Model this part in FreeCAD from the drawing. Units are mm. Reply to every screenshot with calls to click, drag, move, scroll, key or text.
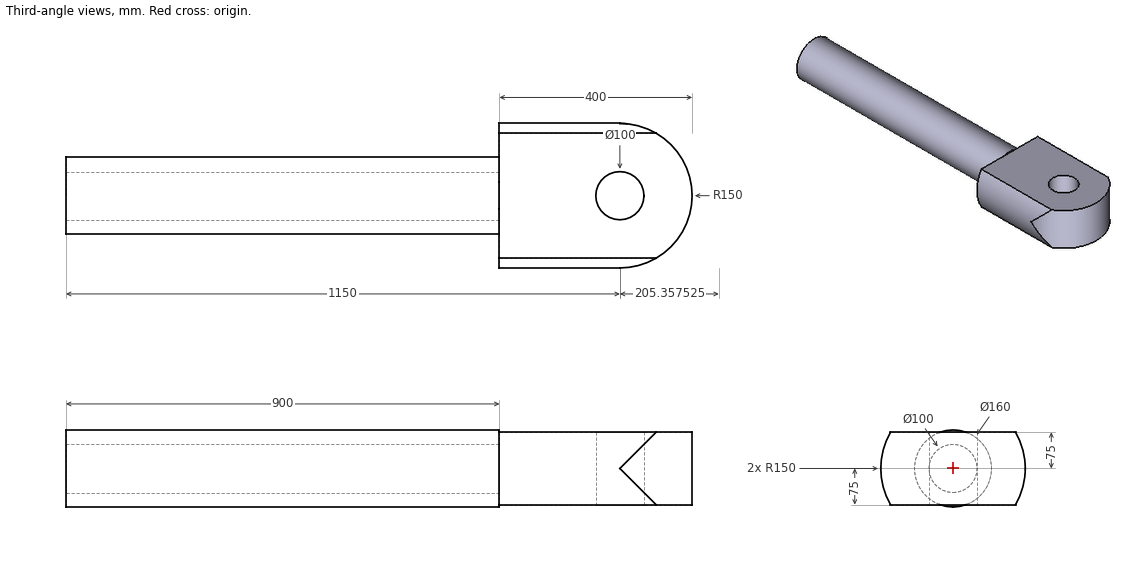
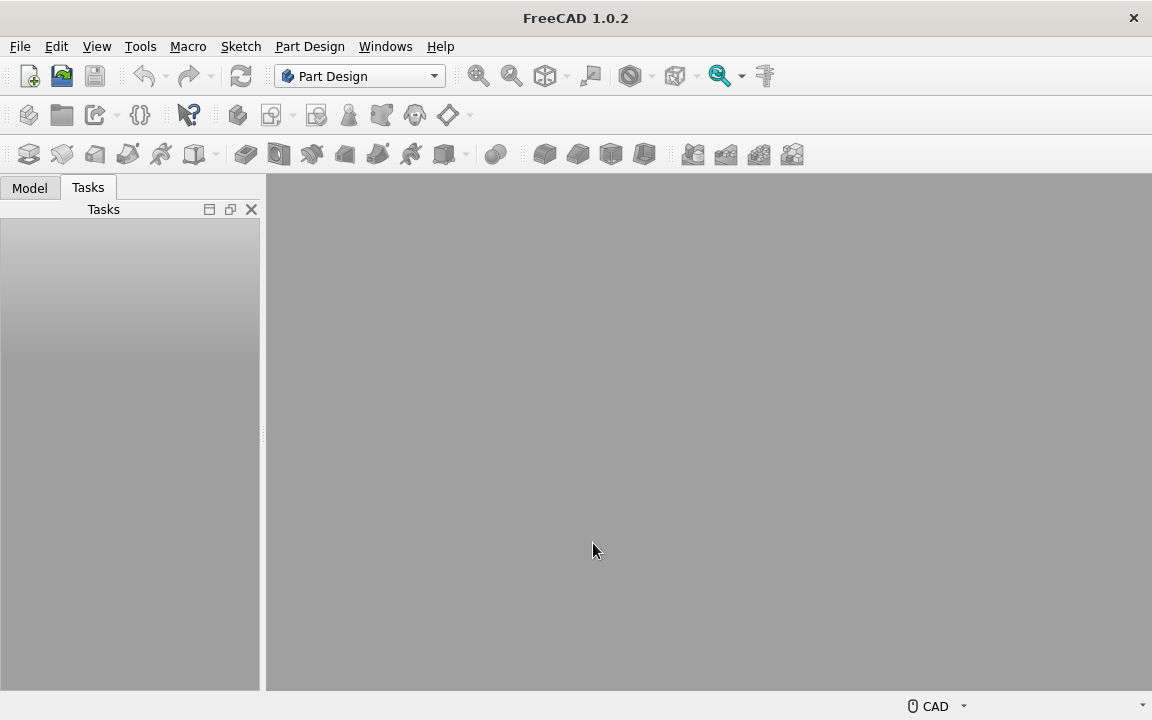
key(ctrl+n)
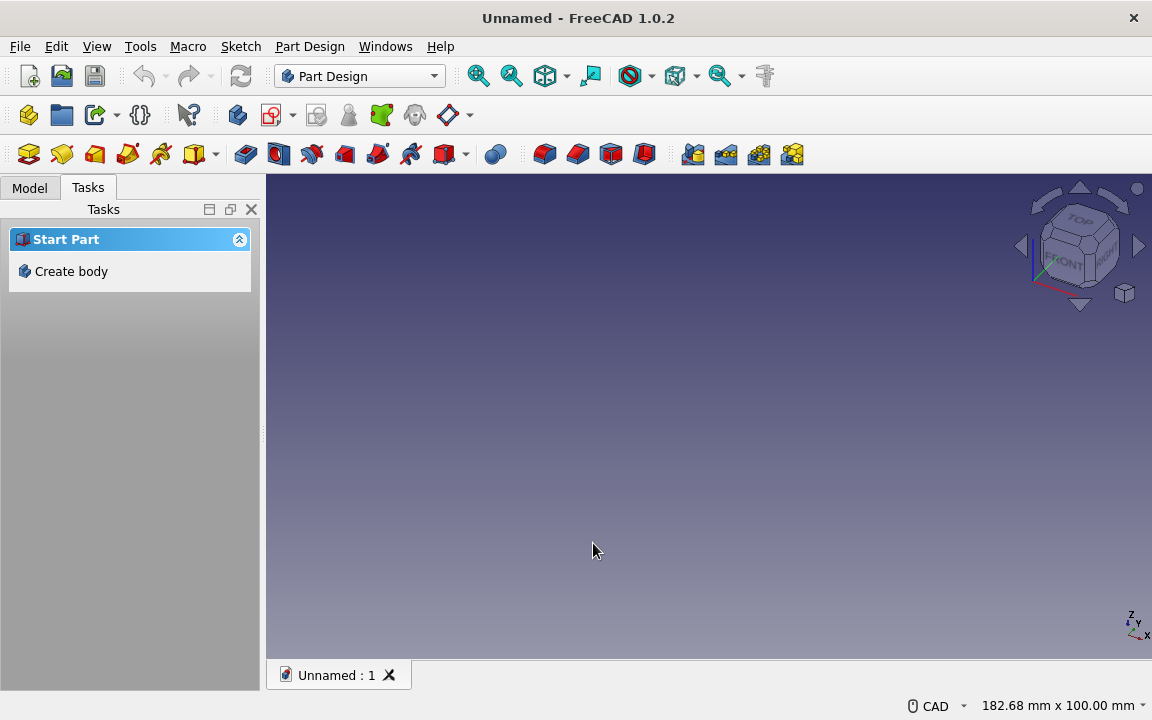
click(238, 116)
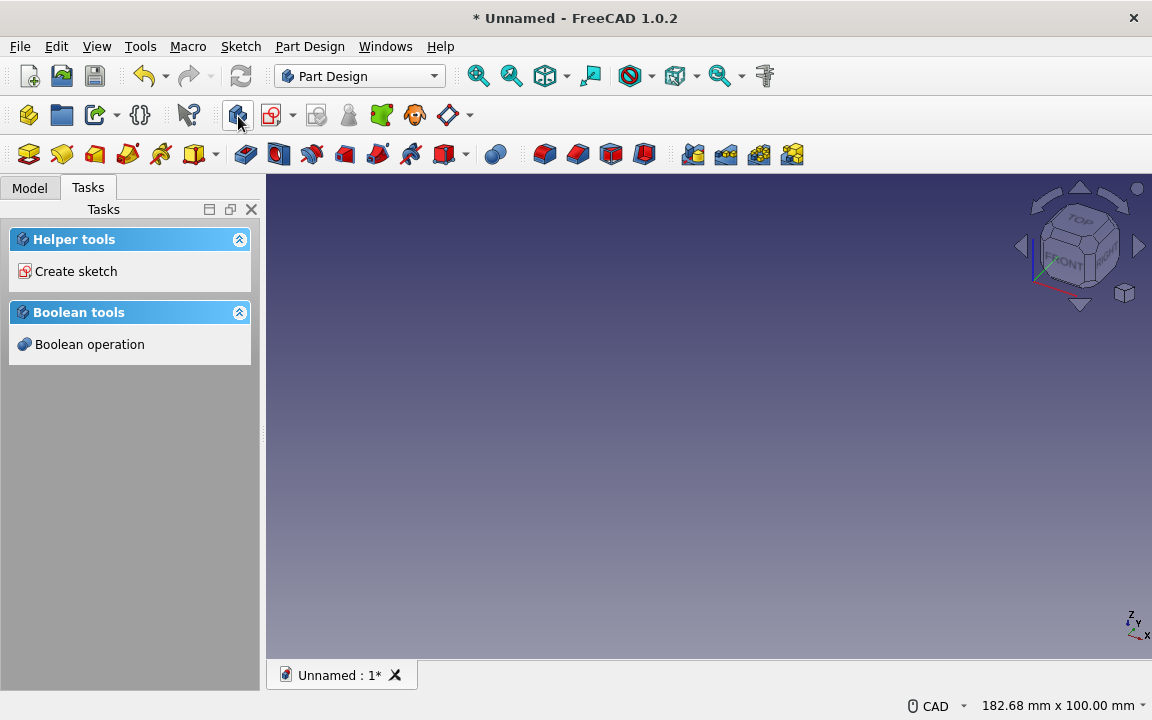
click(30, 188)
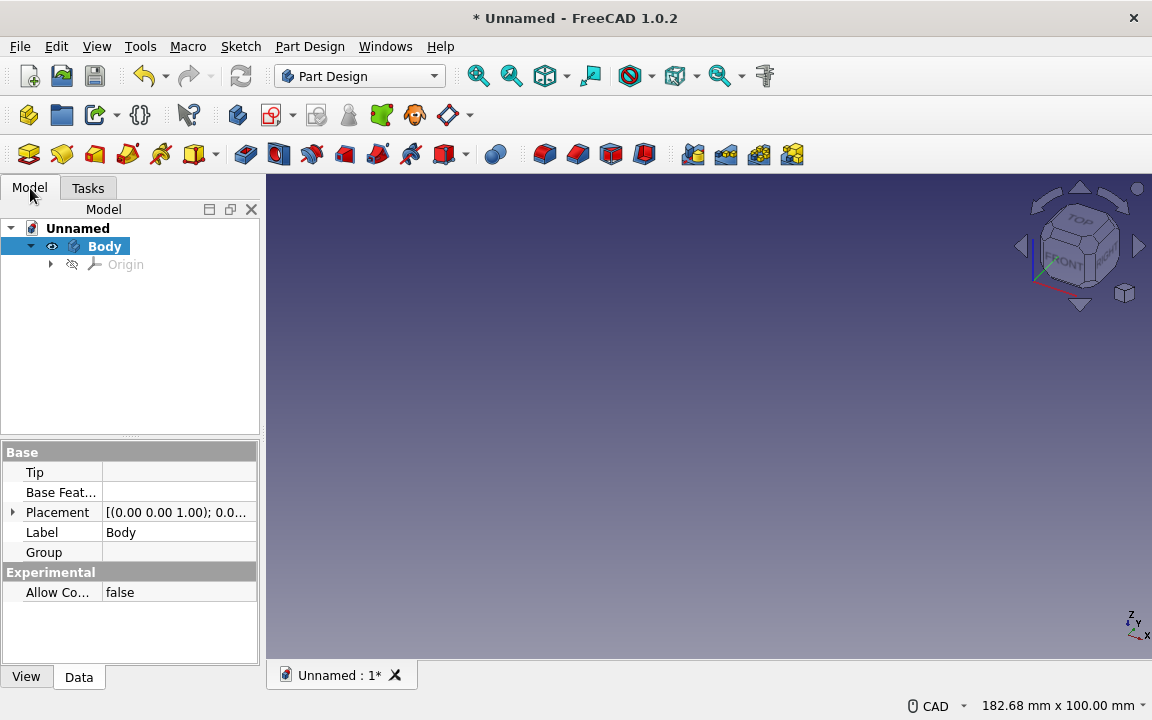
click(51, 264)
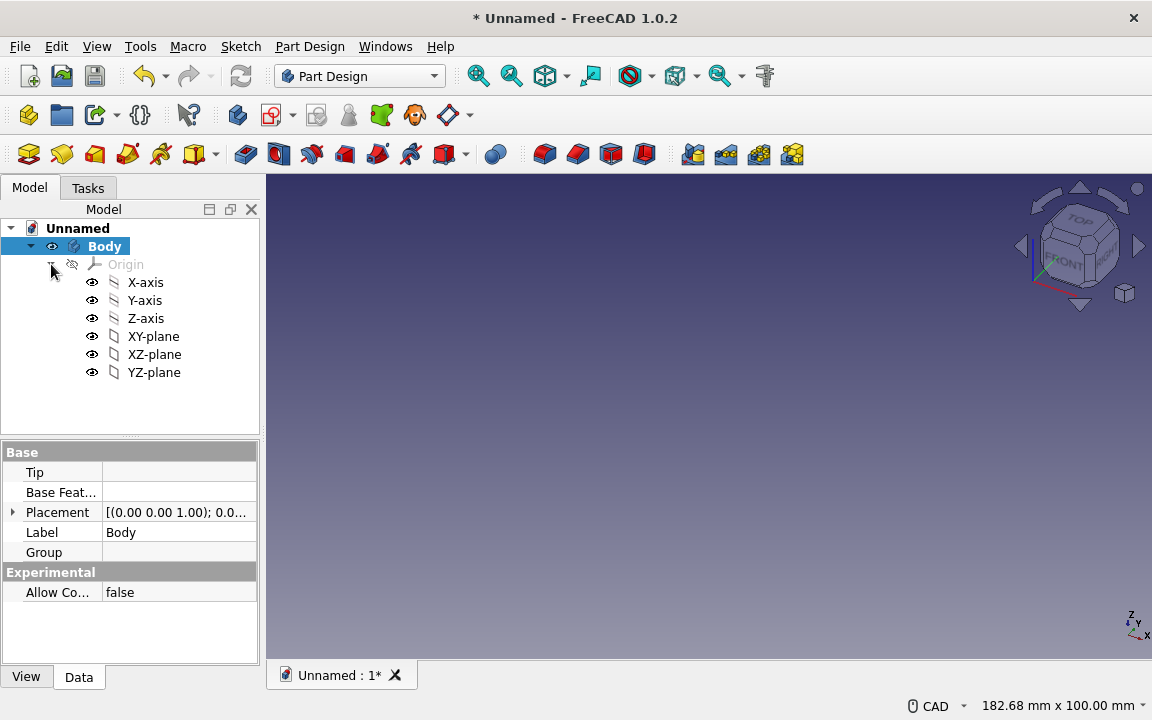
click(137, 372)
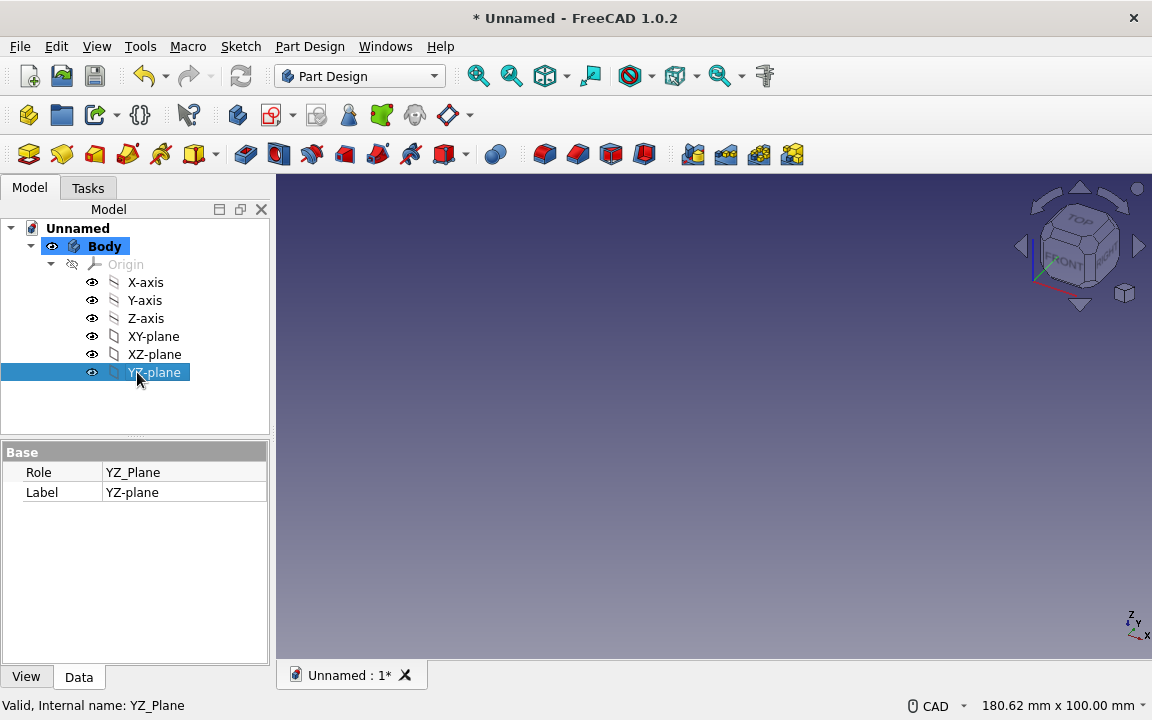
click(448, 116)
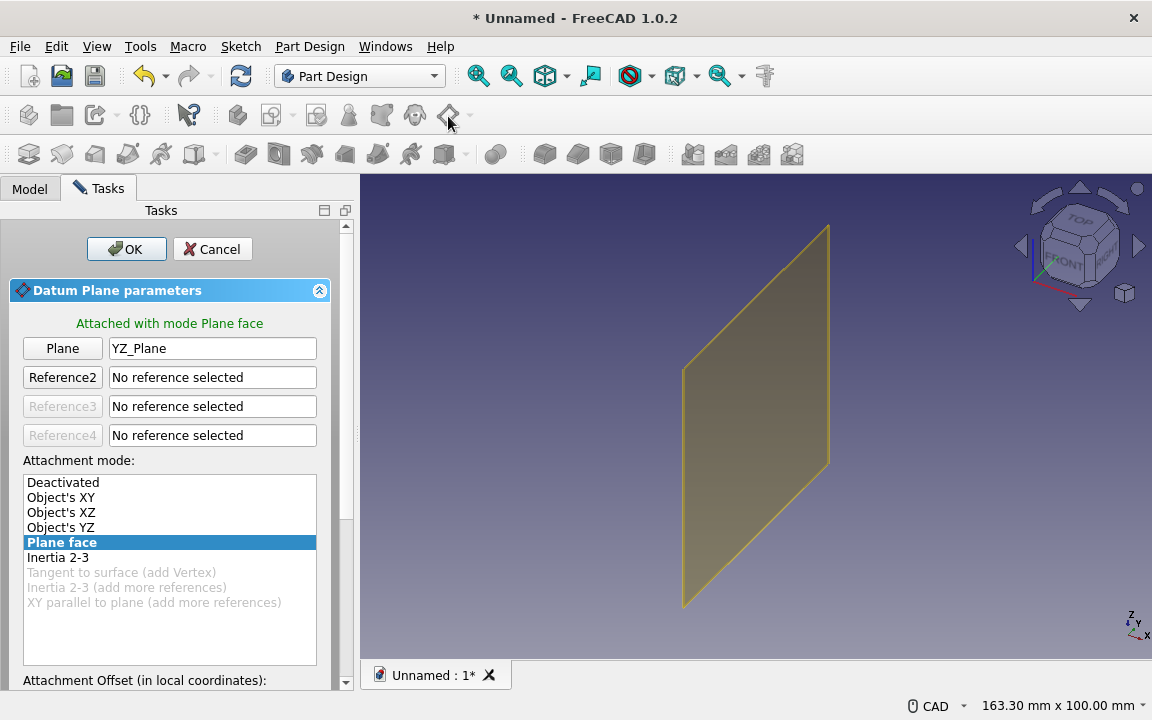
scroll(346, 455, down, 3)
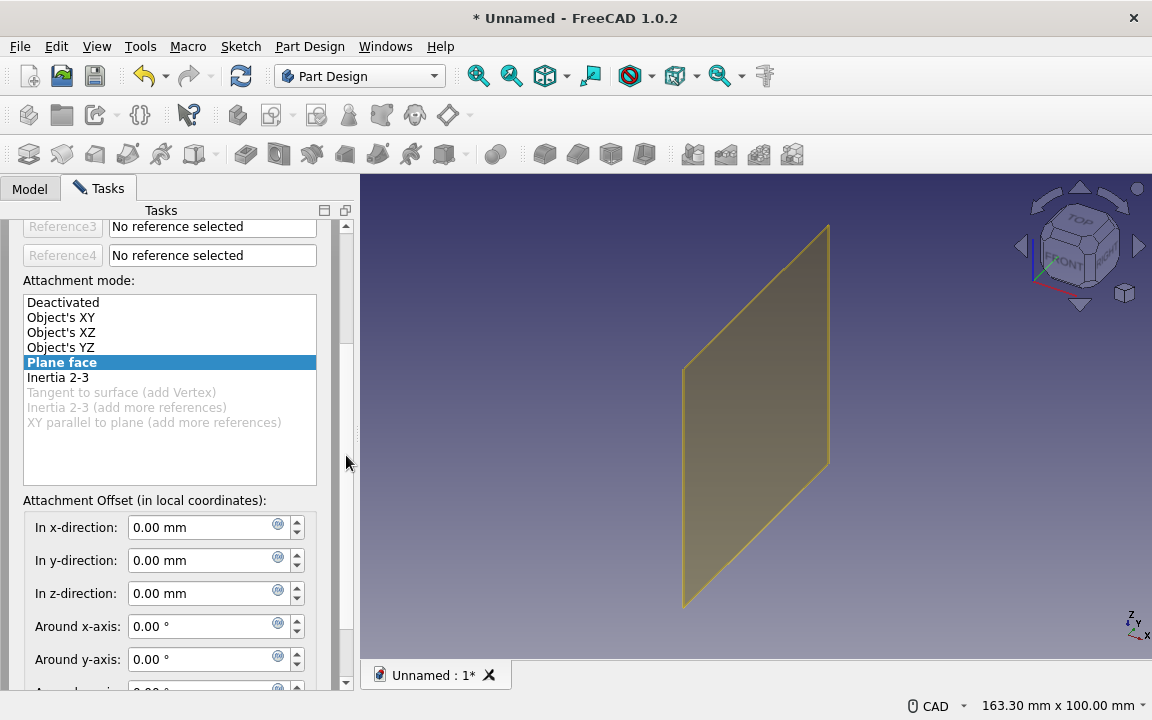
triple_click(210, 594)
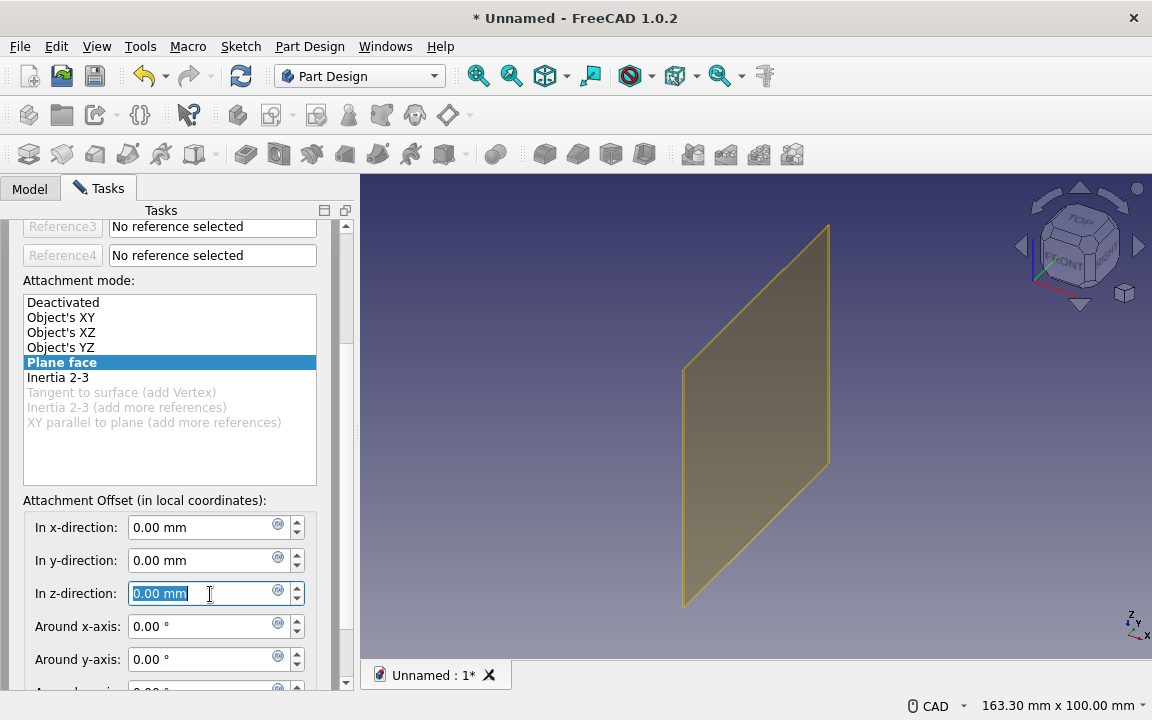
text(100)
key(Tab)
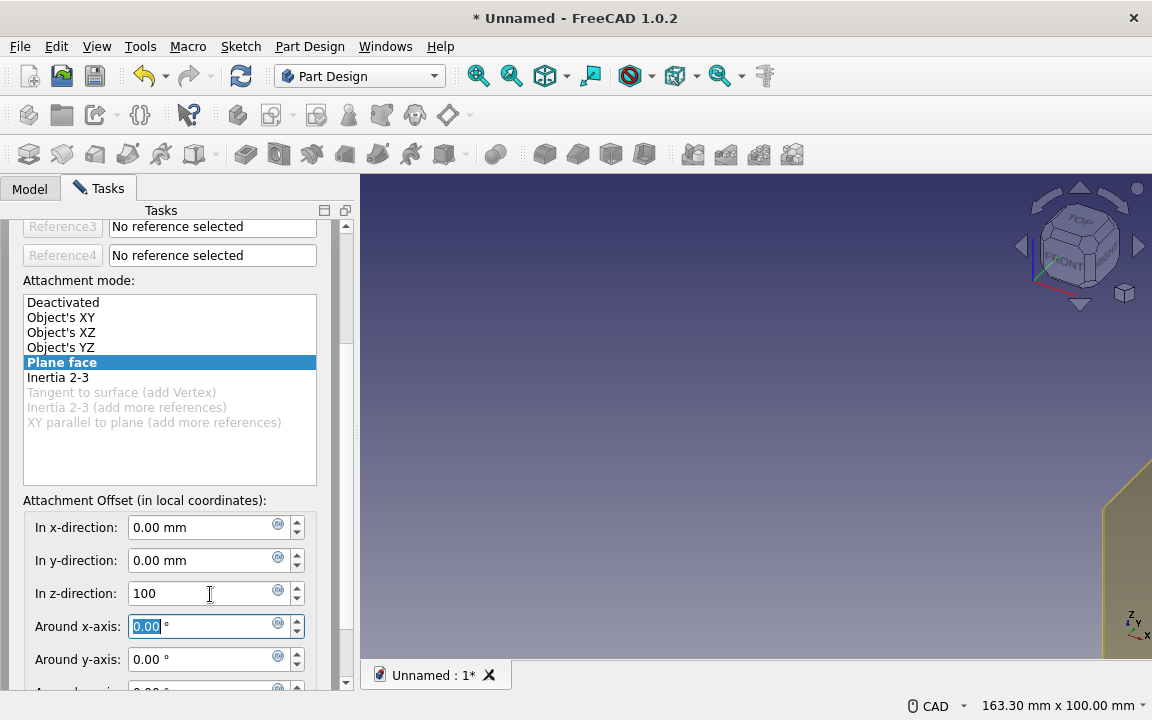
scroll(346, 455, up, 4)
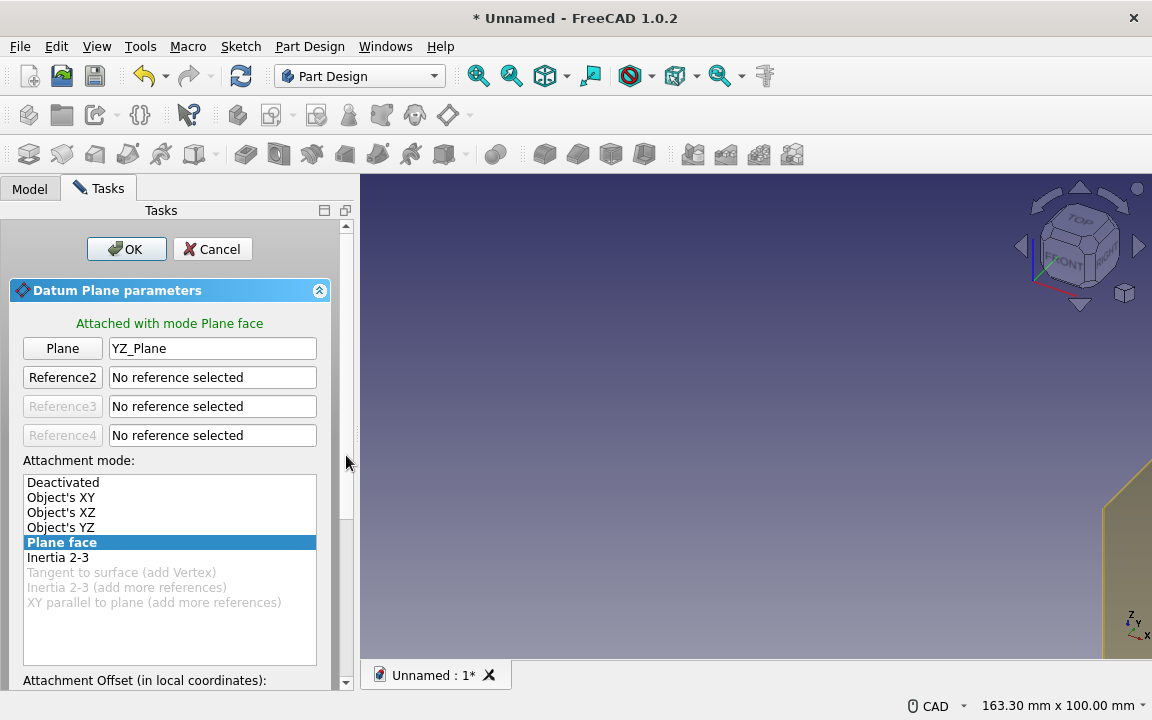
click(127, 249)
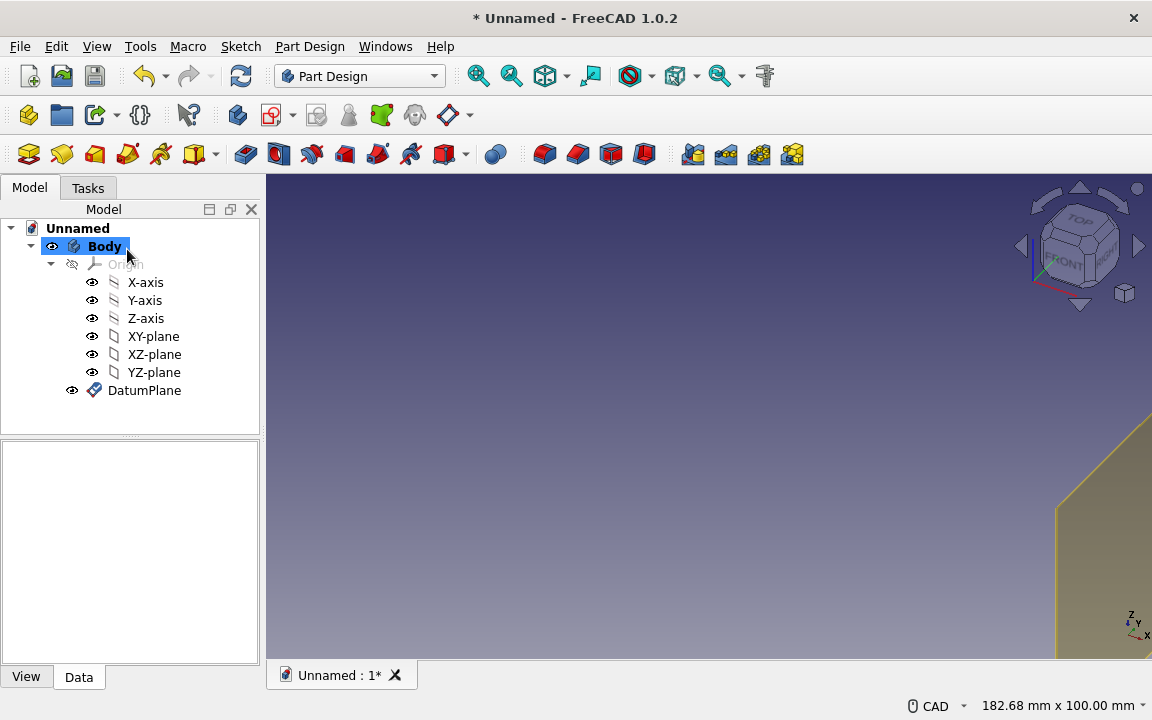
click(117, 390)